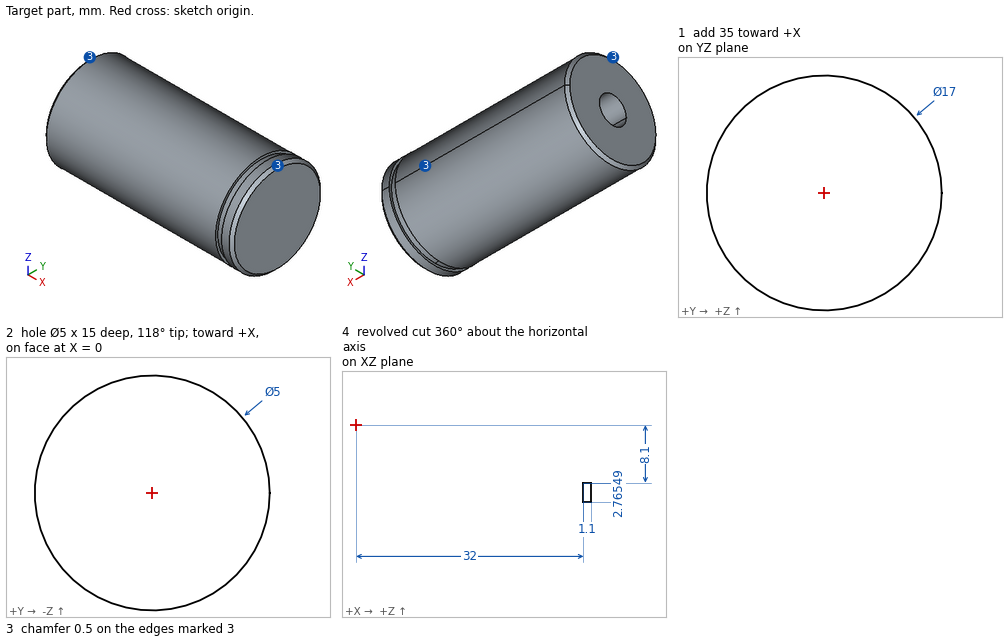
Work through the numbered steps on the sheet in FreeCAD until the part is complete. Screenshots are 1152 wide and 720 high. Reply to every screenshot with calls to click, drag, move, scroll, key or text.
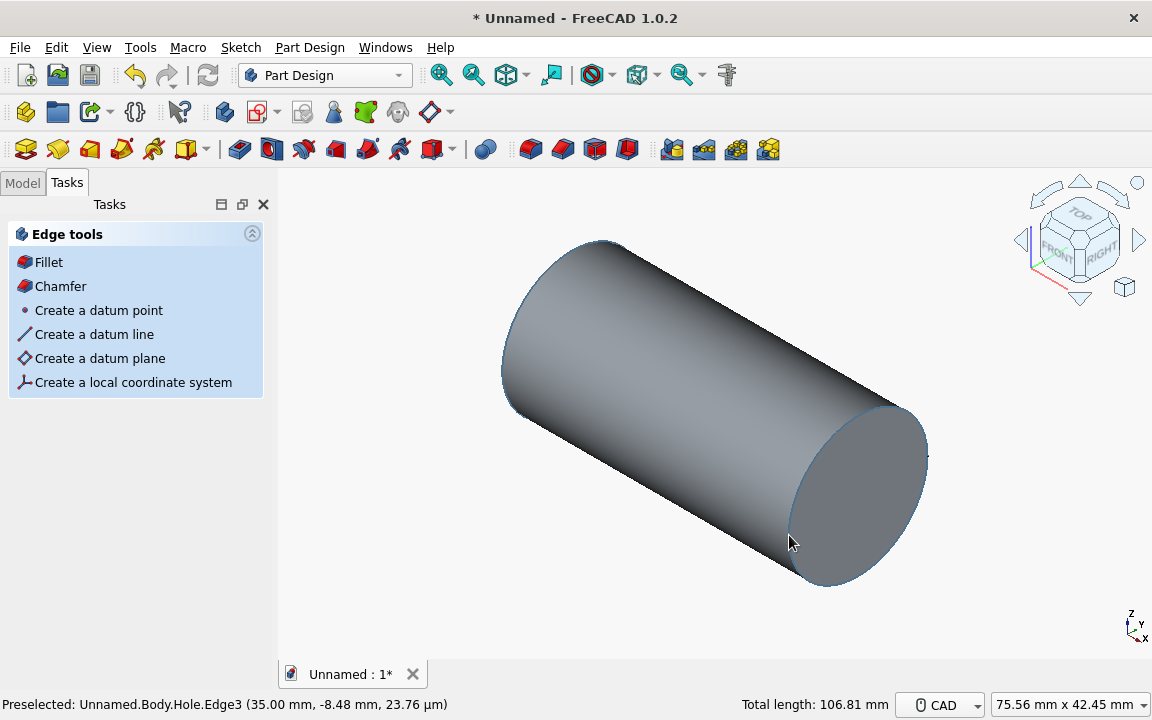
click(564, 150)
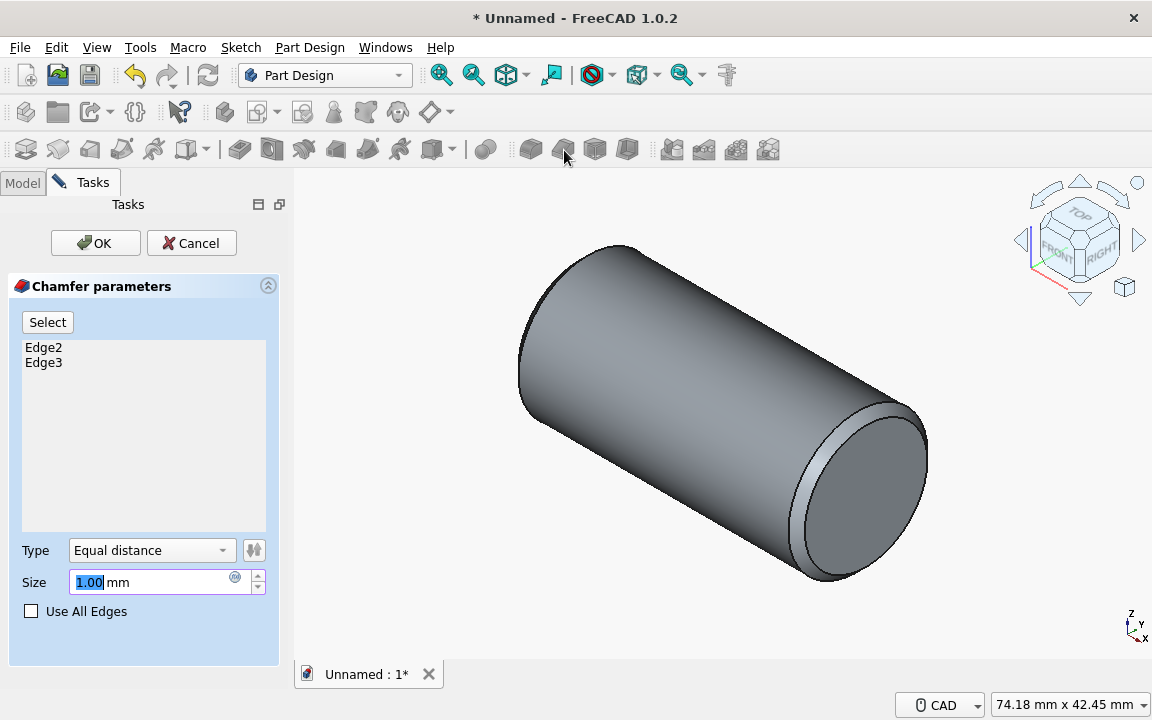
text(0.5)
key(Tab)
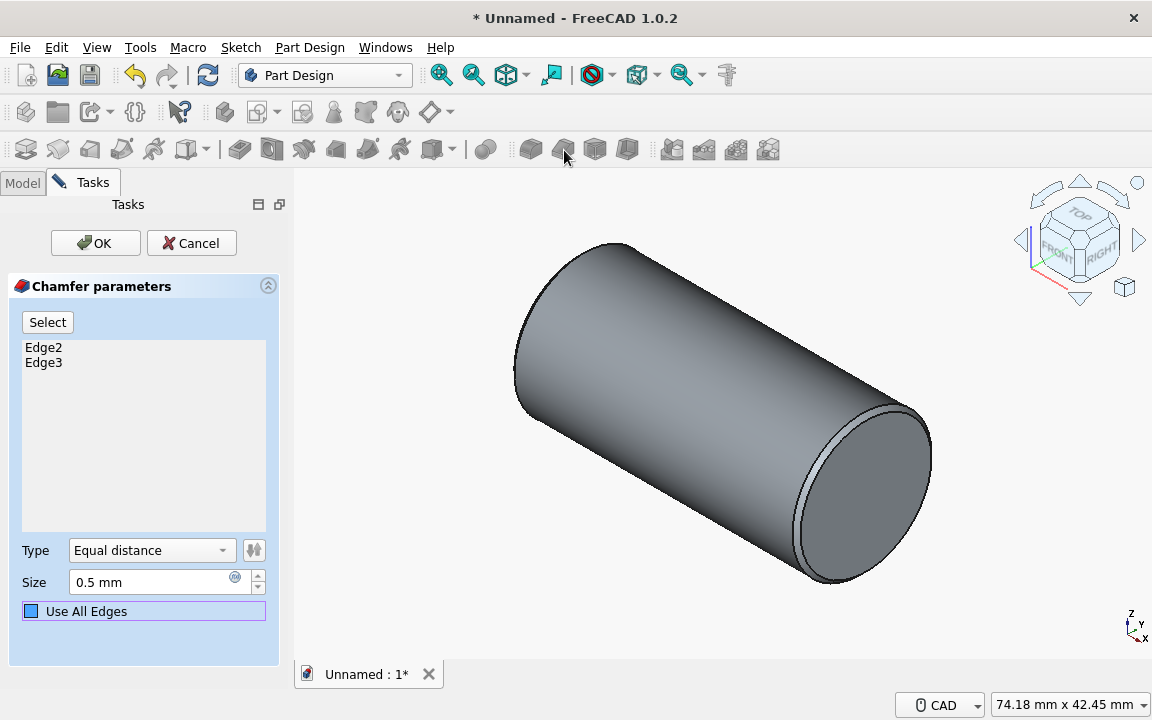
click(96, 243)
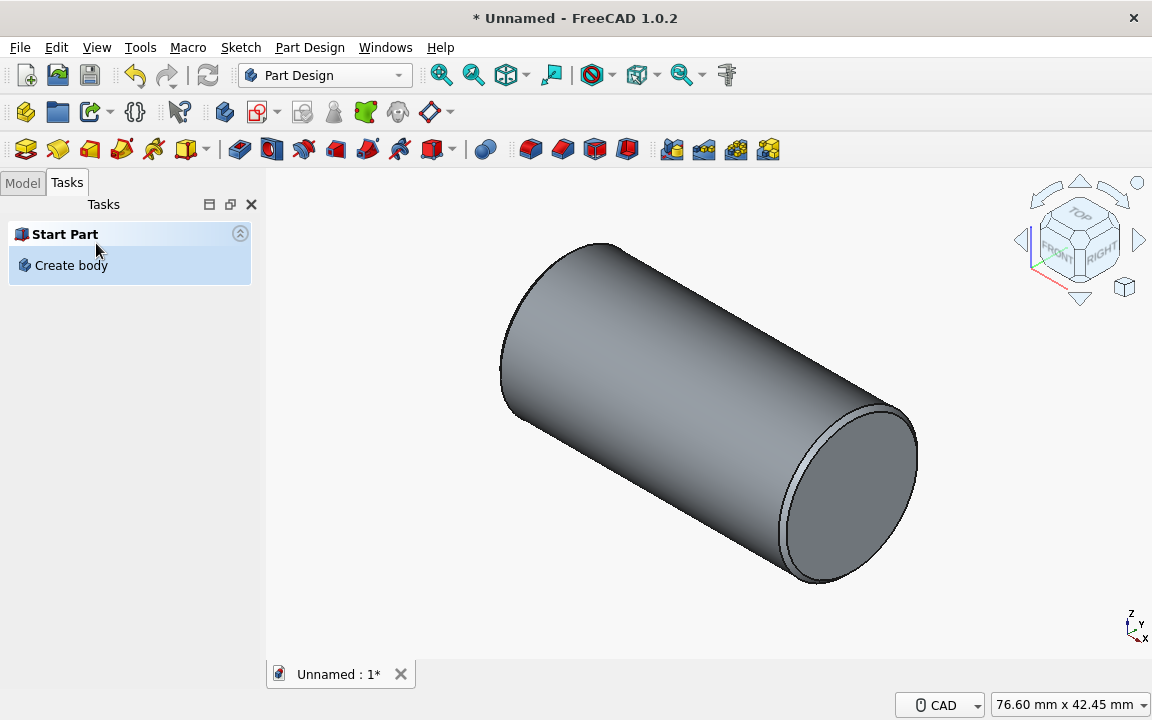
click(258, 112)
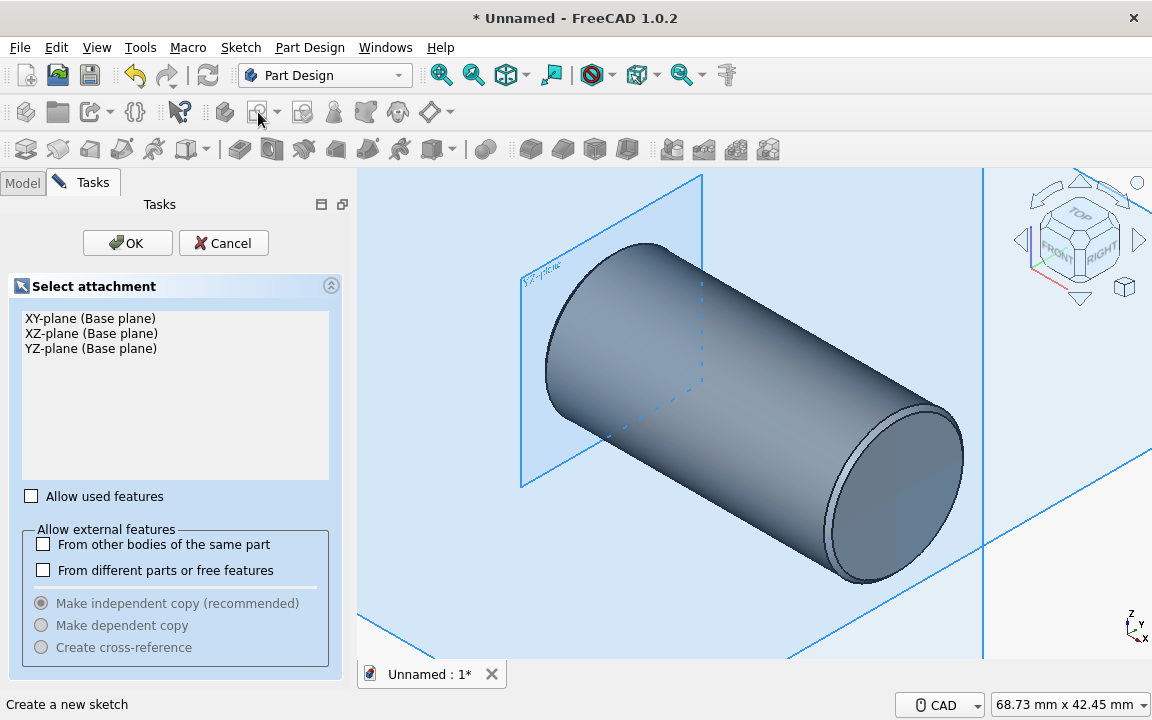
click(82, 334)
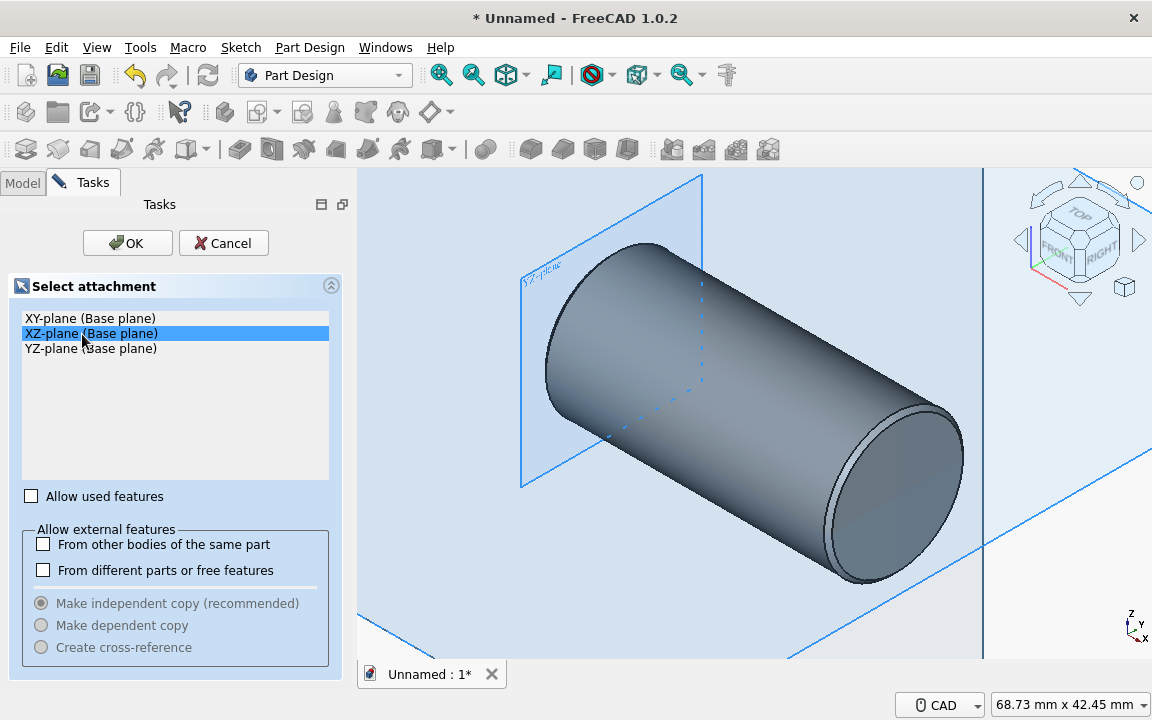
click(128, 243)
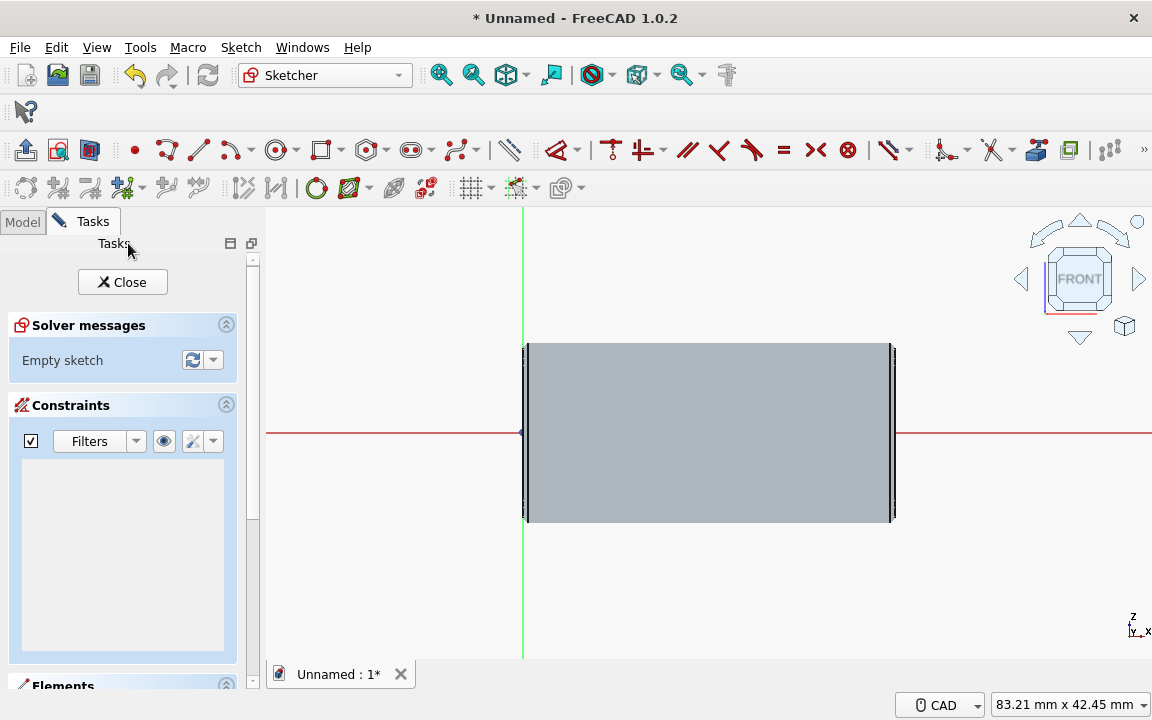
click(90, 150)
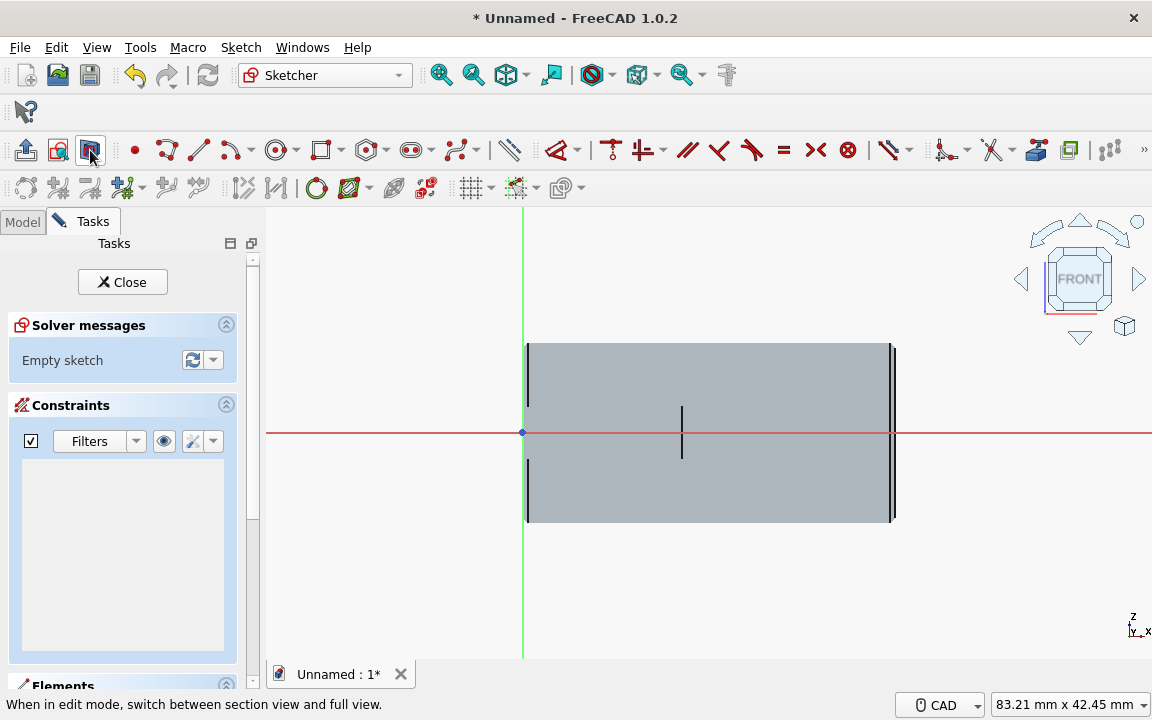
scroll(898, 547, up, 11)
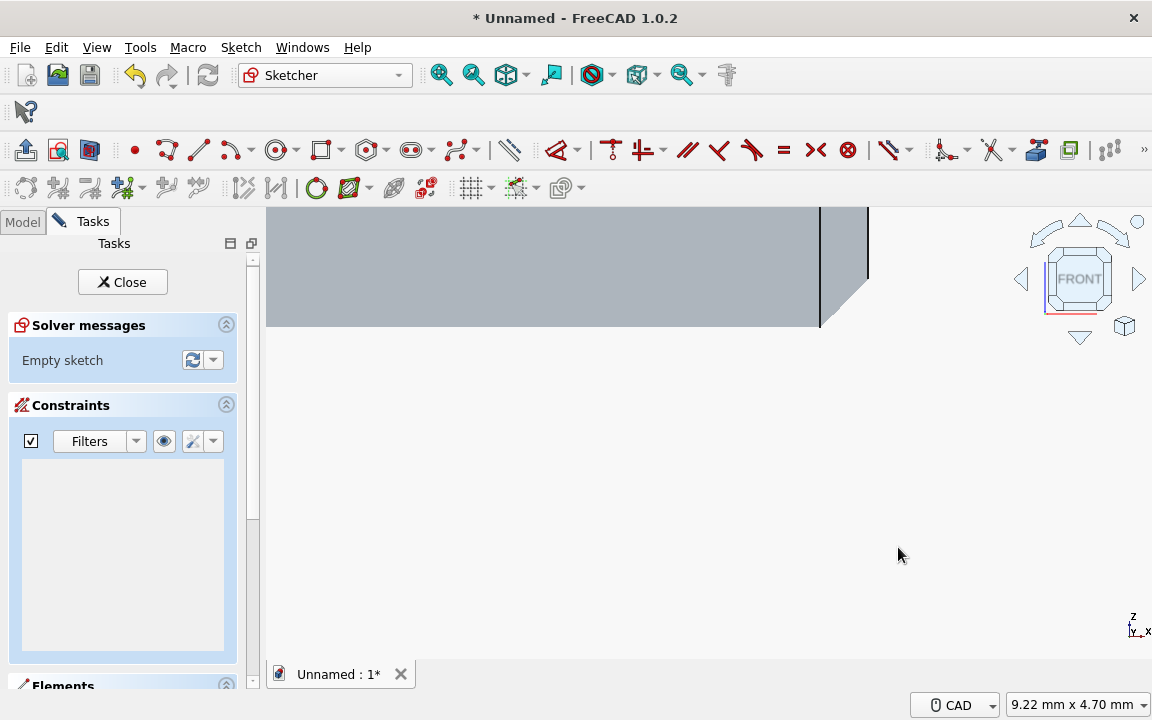
click(322, 150)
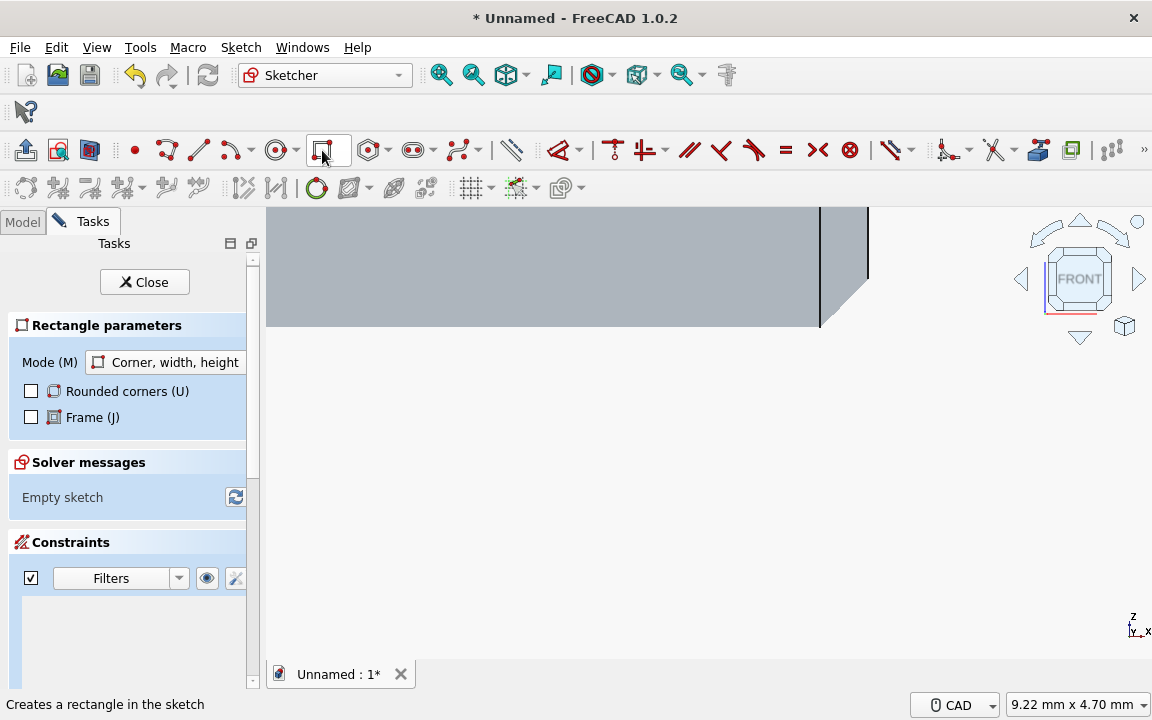
click(580, 291)
click(686, 556)
key(Escape)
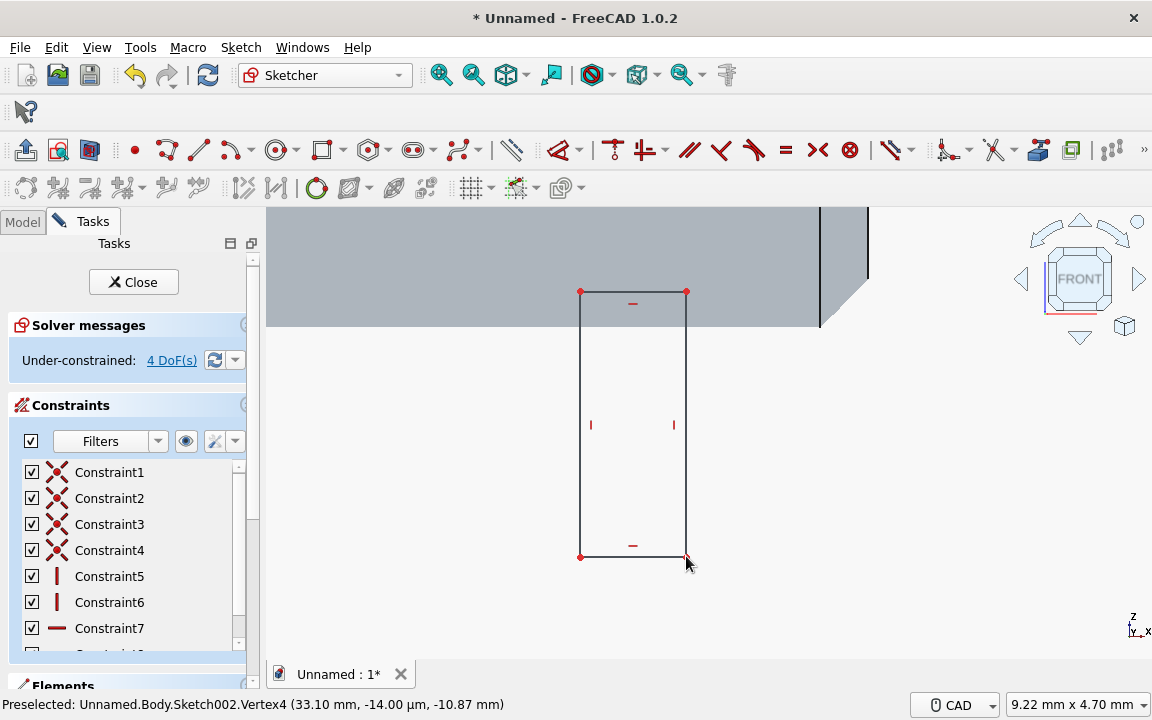
click(558, 150)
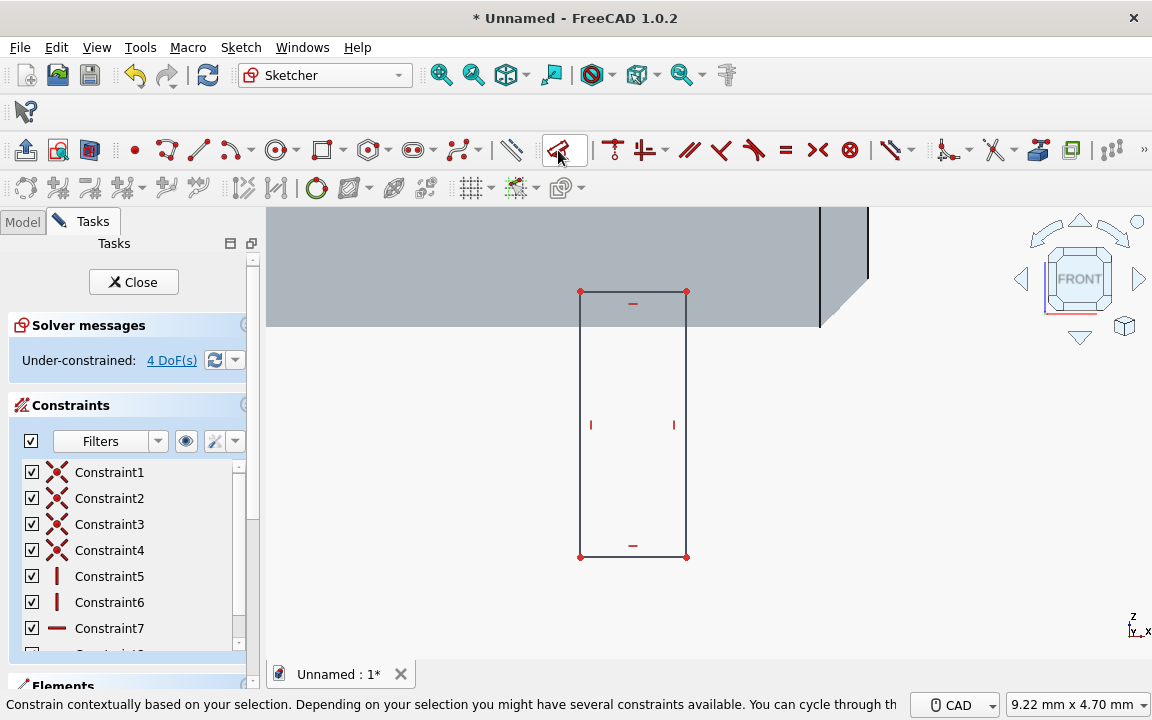
click(612, 557)
click(633, 591)